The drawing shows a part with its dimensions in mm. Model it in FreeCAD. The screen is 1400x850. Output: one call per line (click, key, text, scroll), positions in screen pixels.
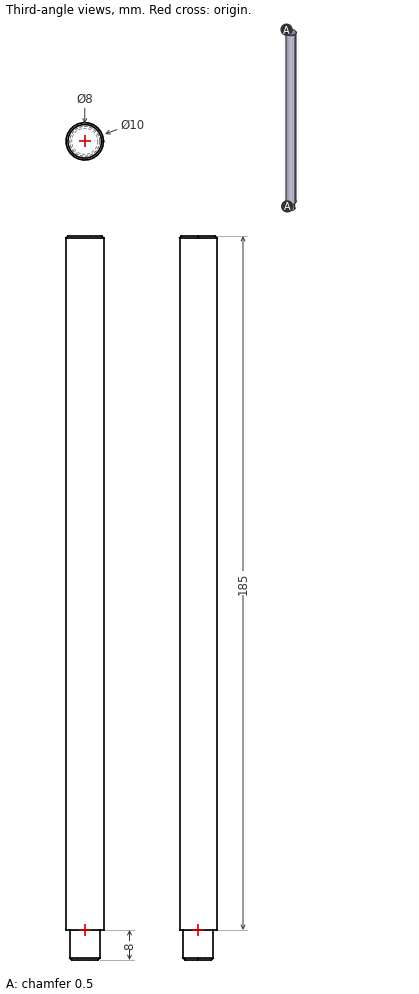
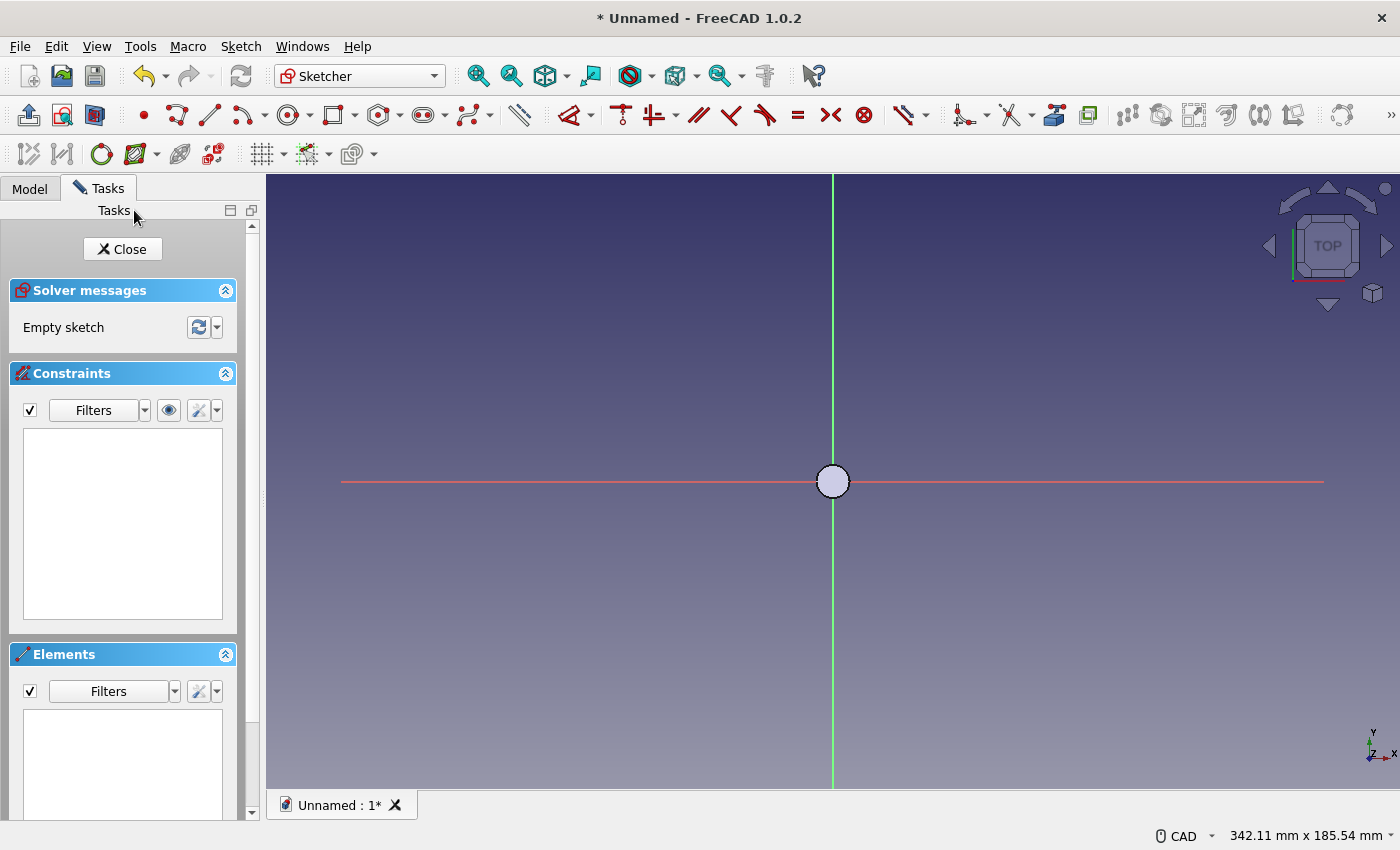
key(q)
key(s)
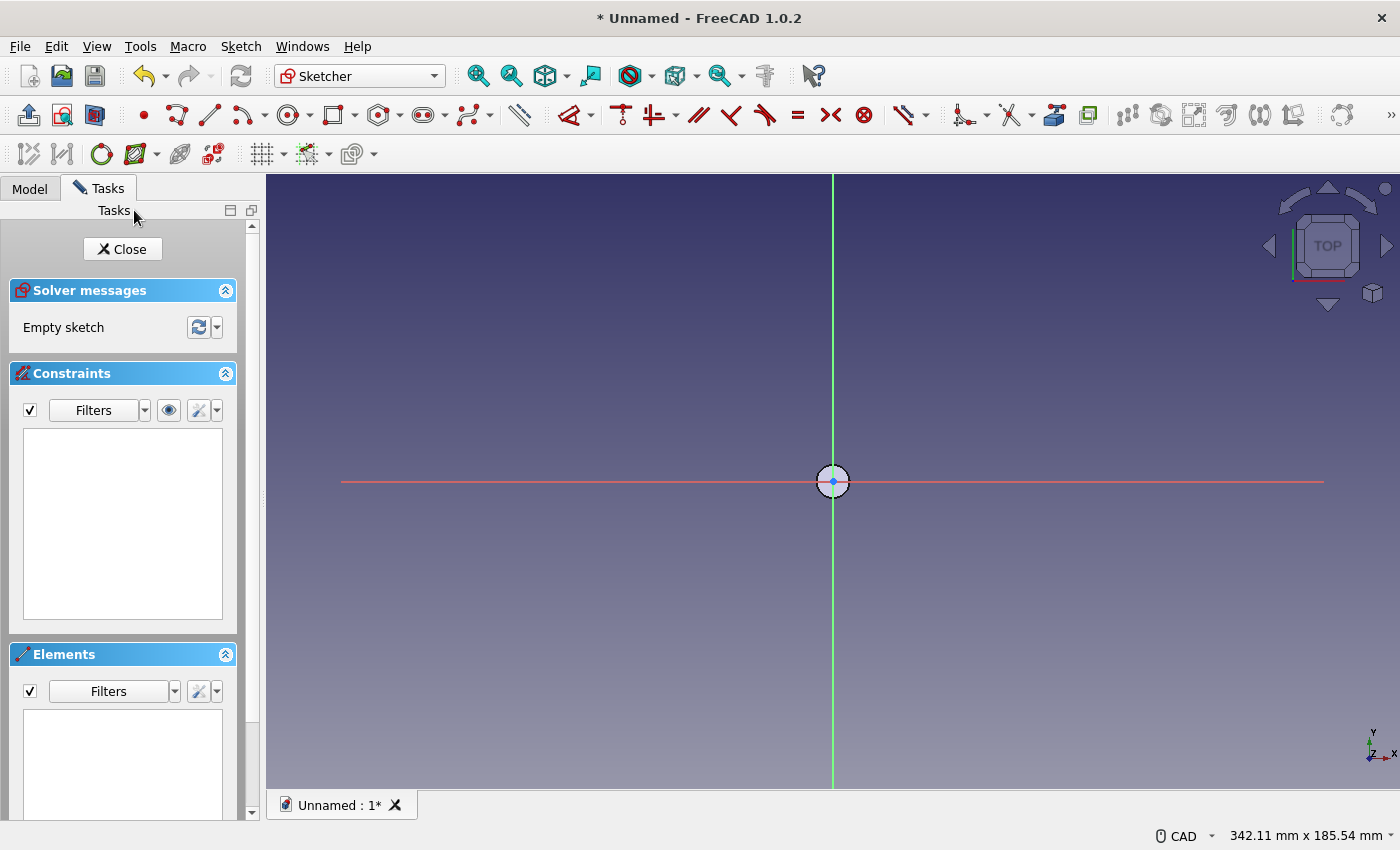
scroll(838, 482, up, 13)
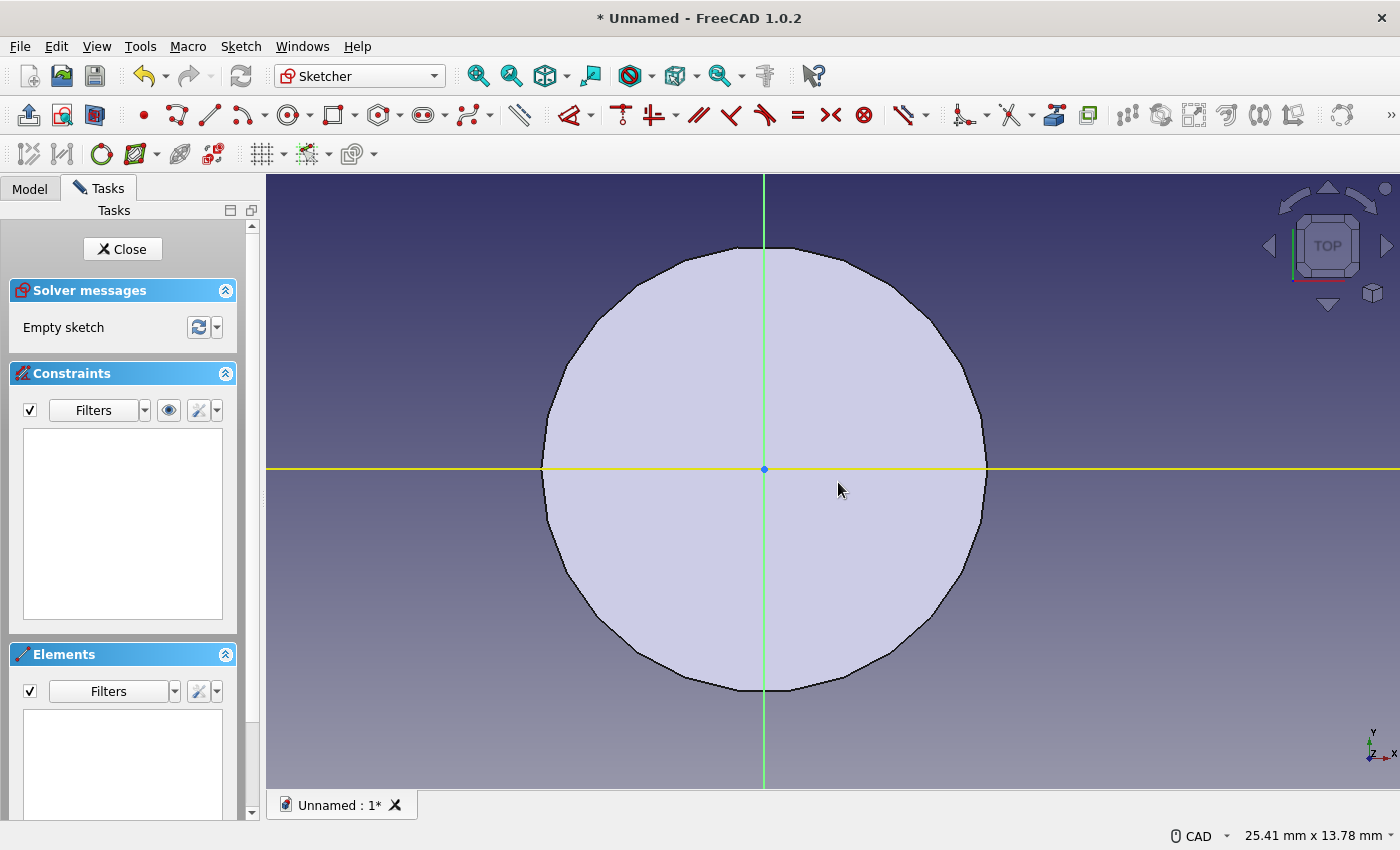
key(g)
key(c)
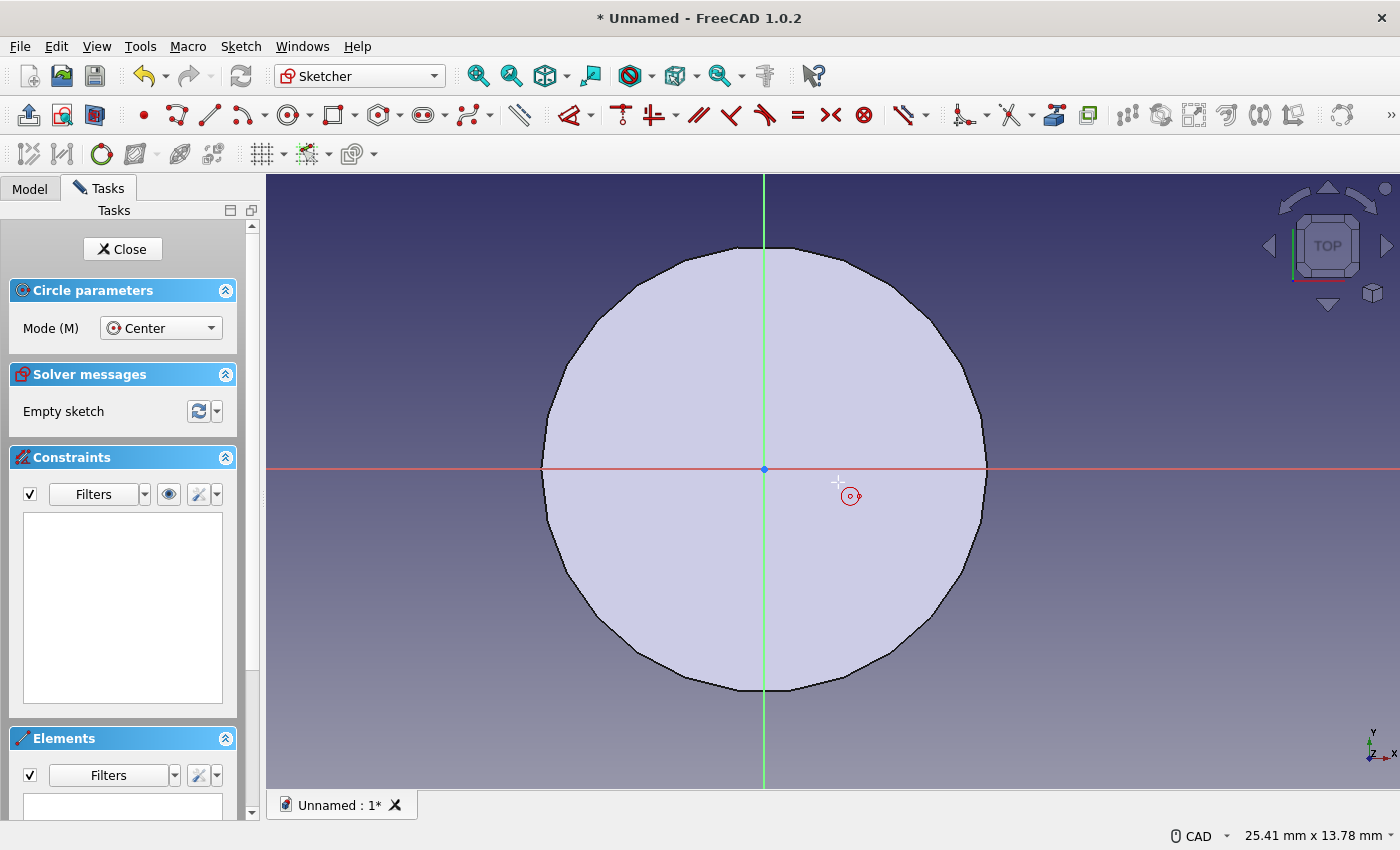
click(764, 469)
click(891, 343)
key(Escape)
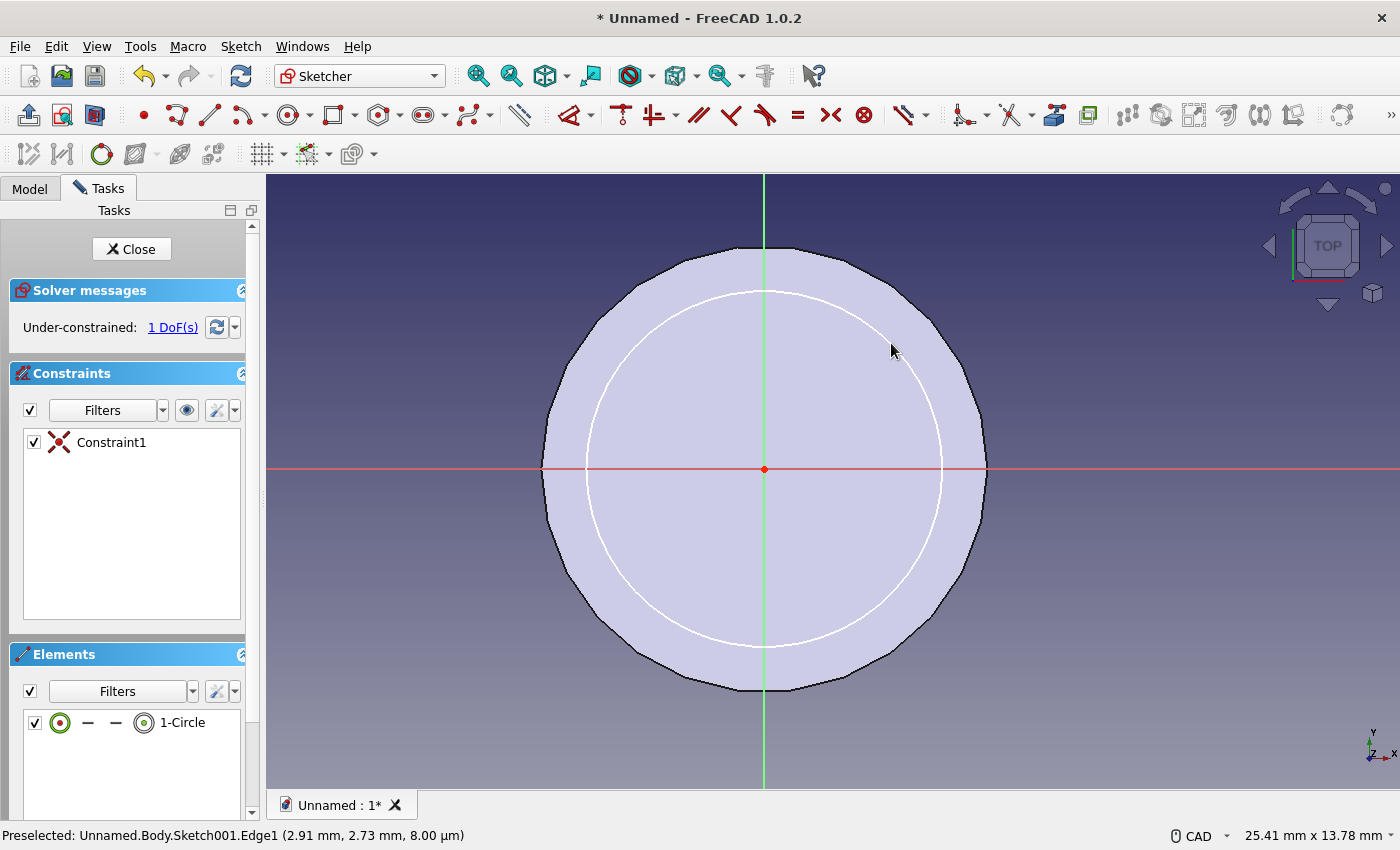
click(890, 343)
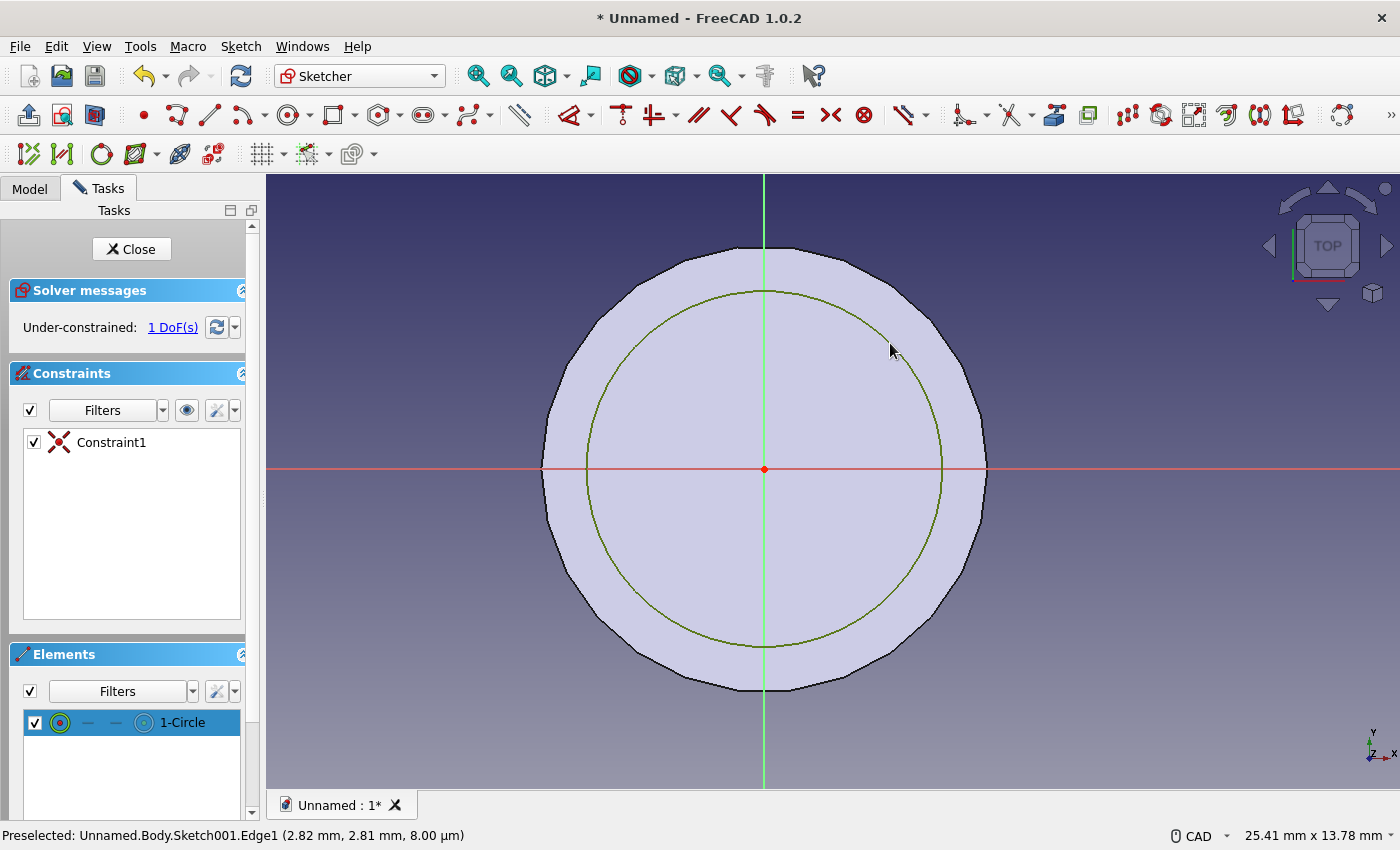
key(k)
key(o)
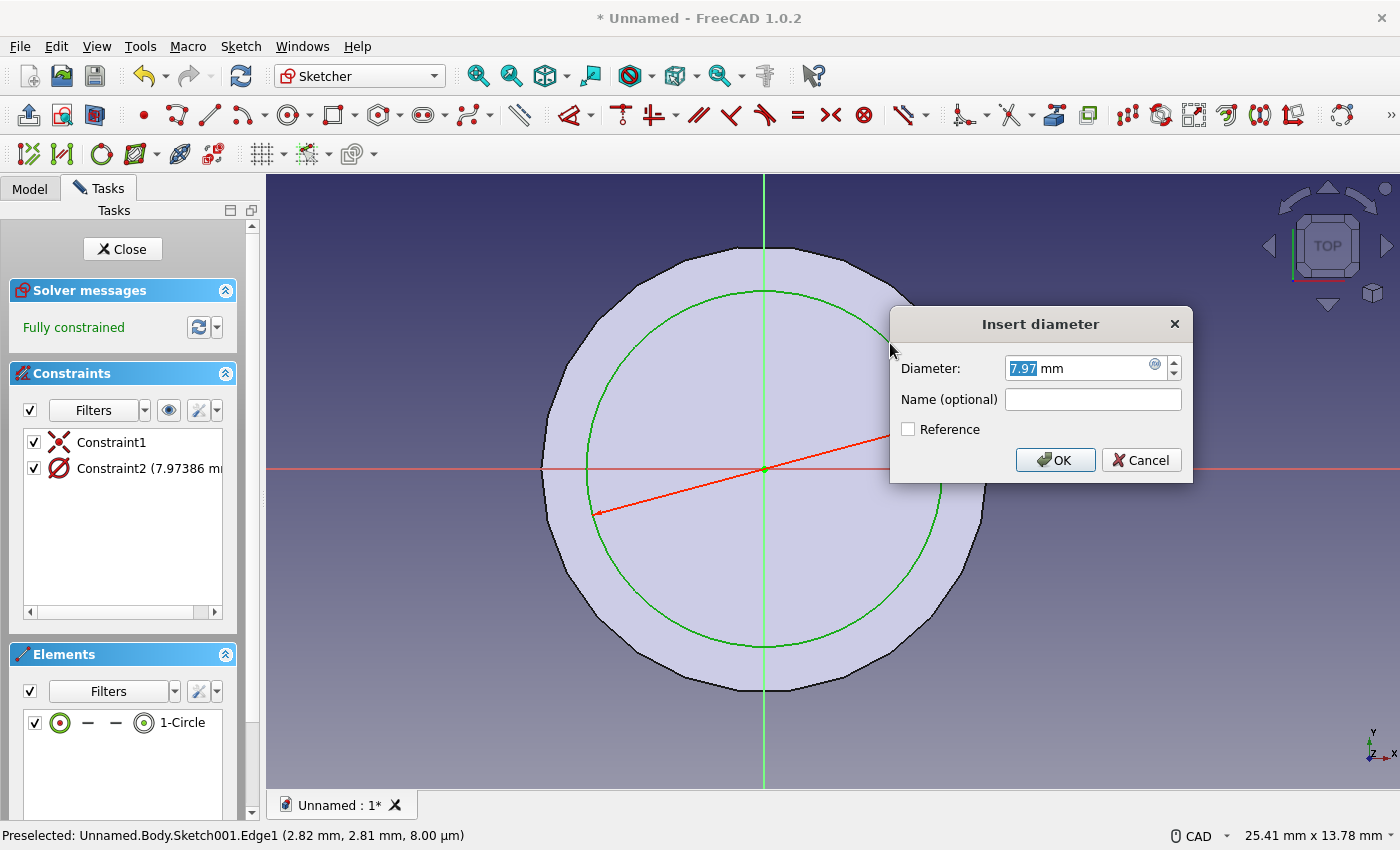
text(8)
key(Return)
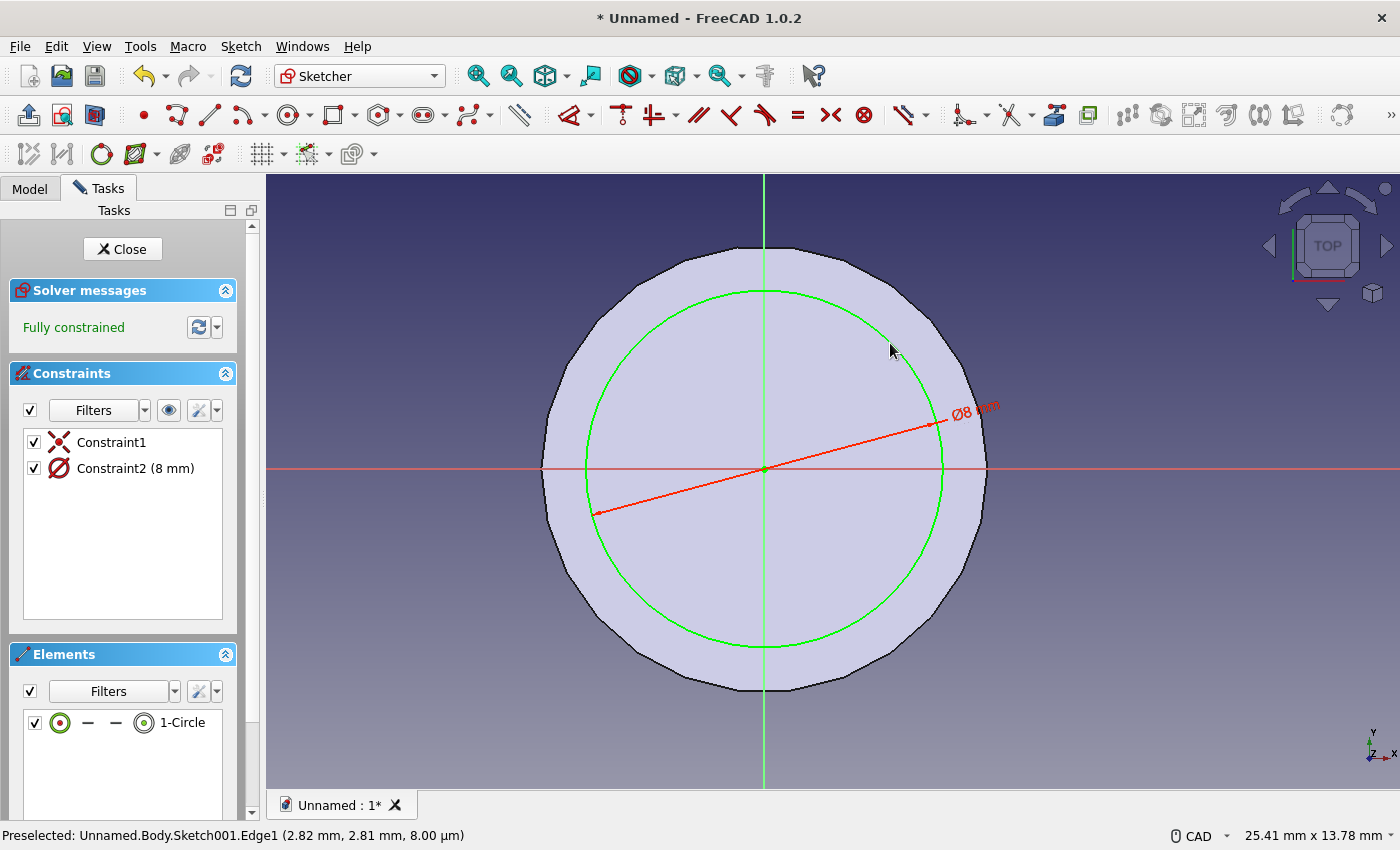
click(123, 249)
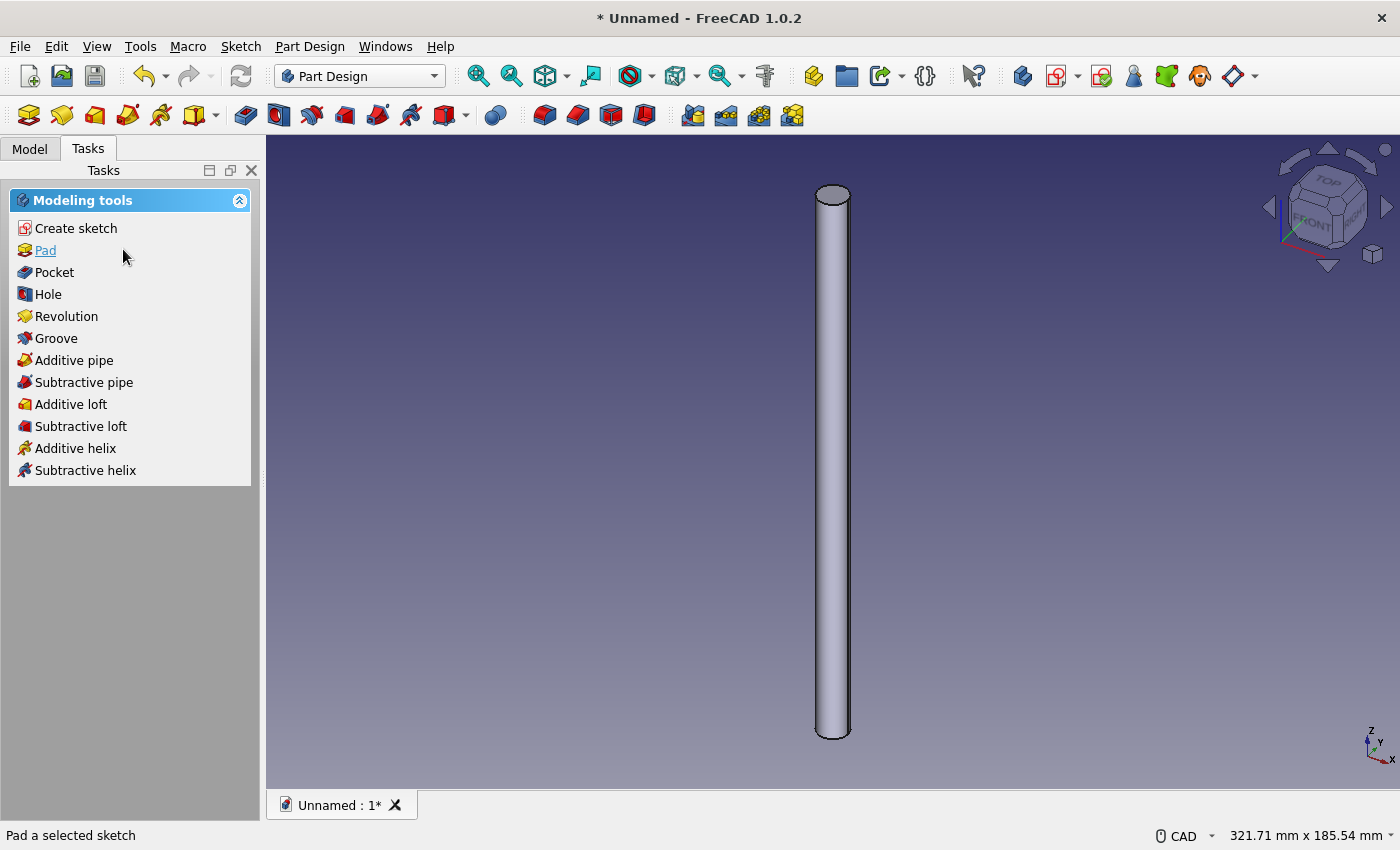
click(29, 116)